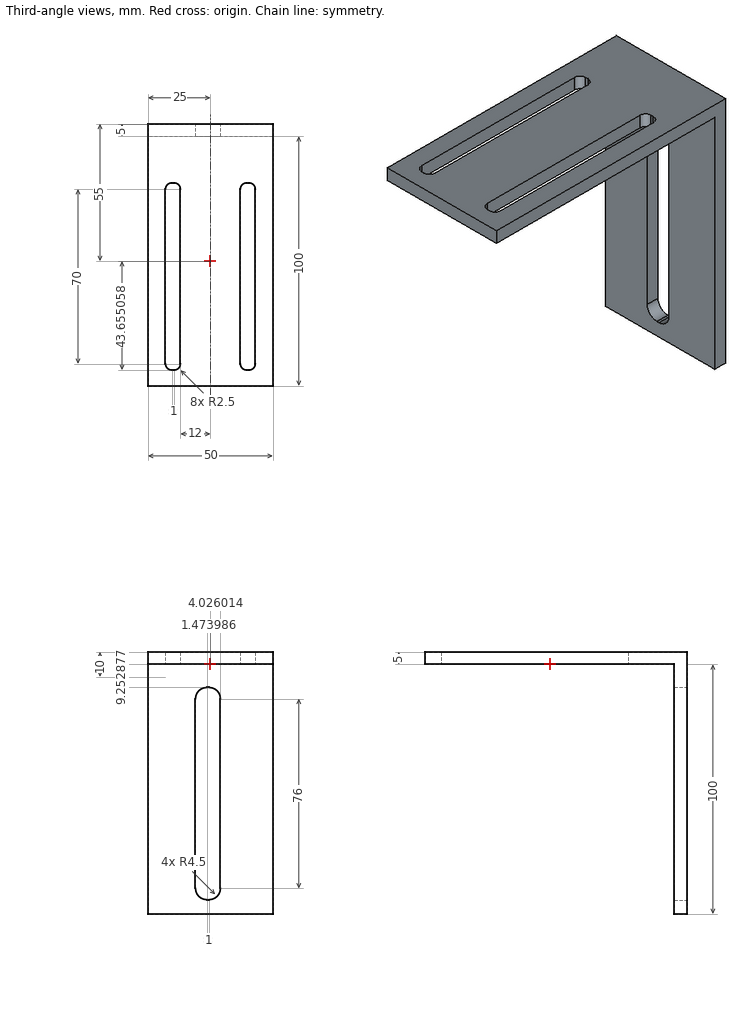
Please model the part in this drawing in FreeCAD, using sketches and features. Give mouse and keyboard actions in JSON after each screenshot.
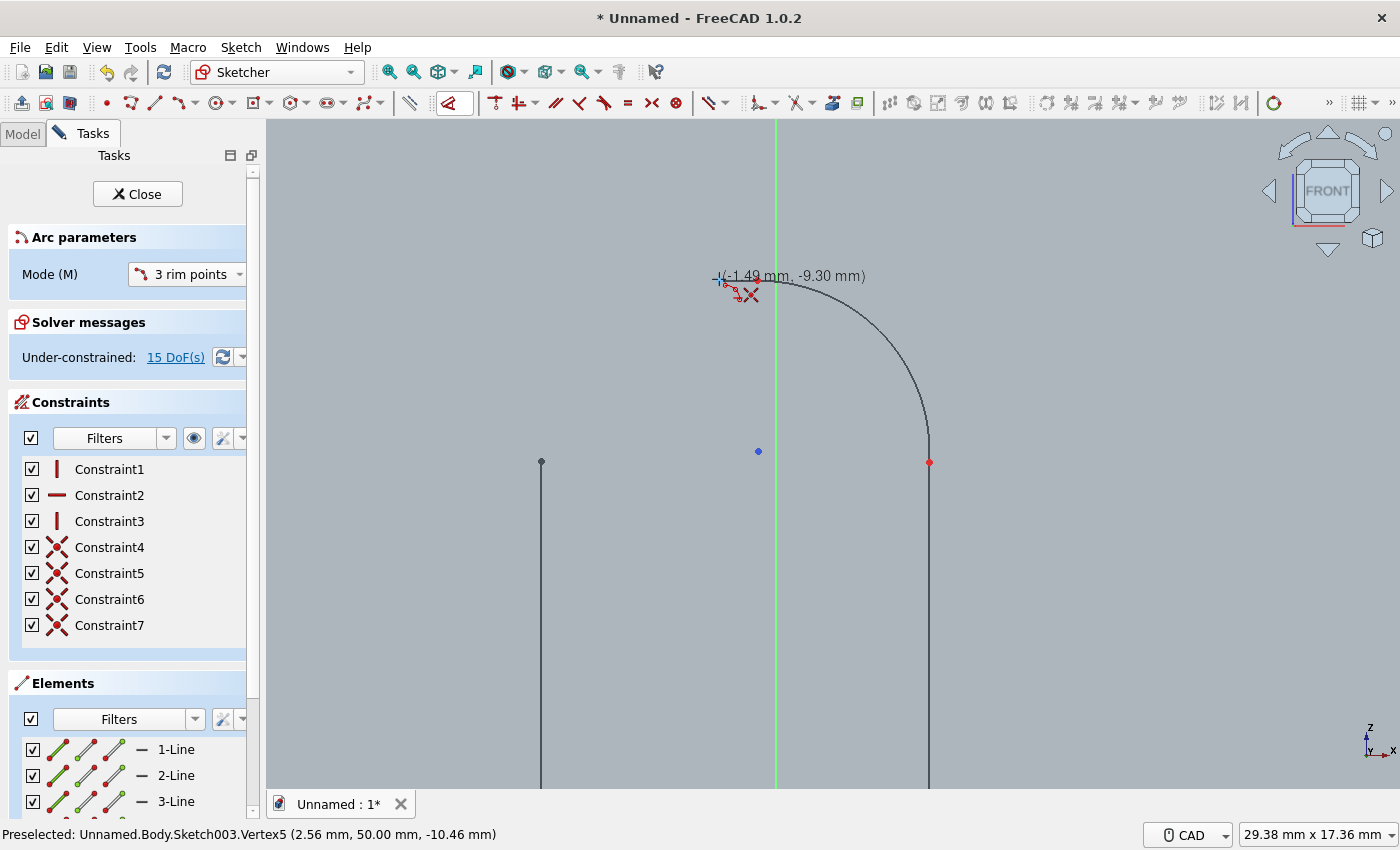
{"action": "left_click", "coordinate": [719, 281]}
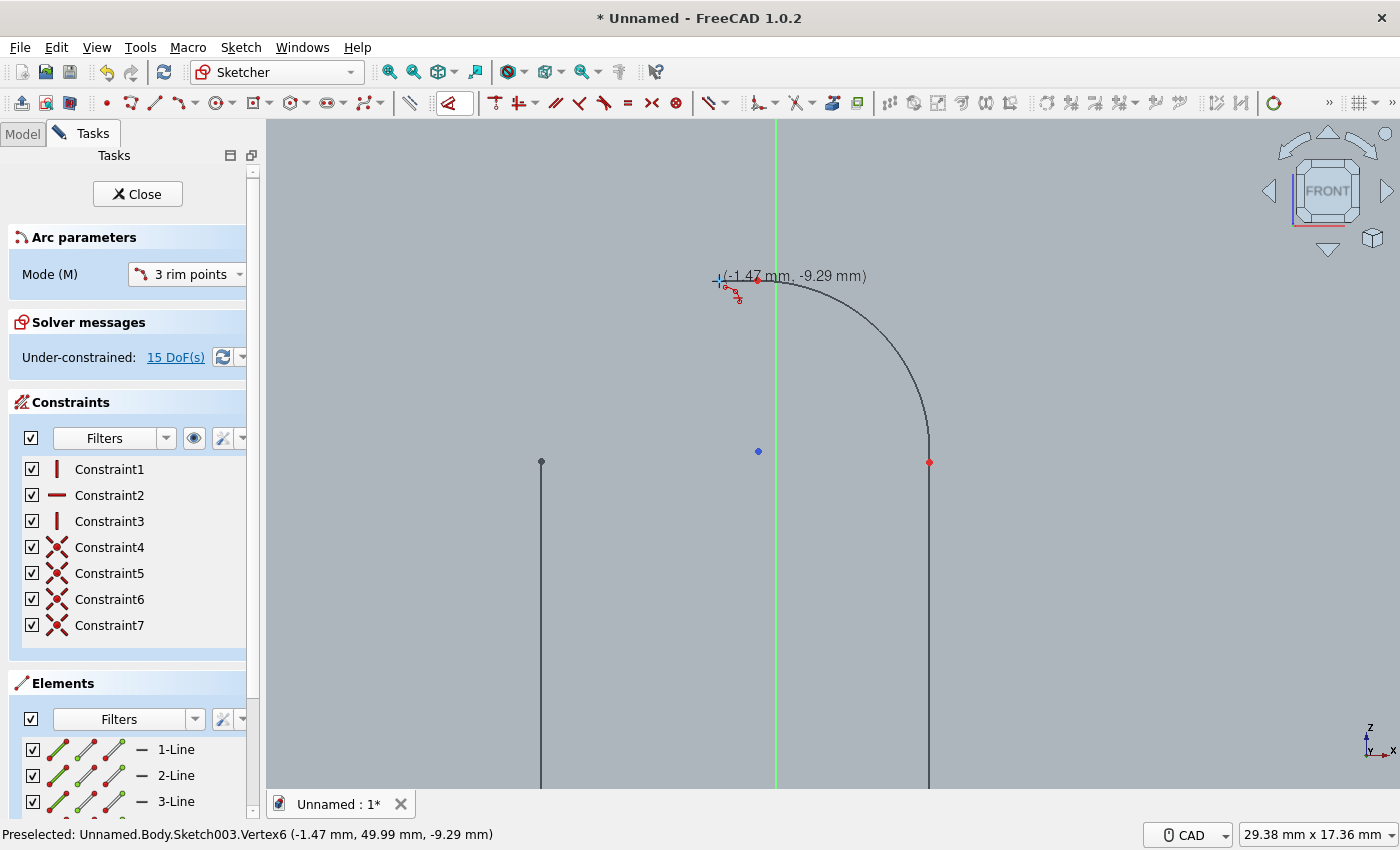
{"action": "scroll", "coordinate": [768, 294], "scroll_direction": "down", "scroll_amount": 11}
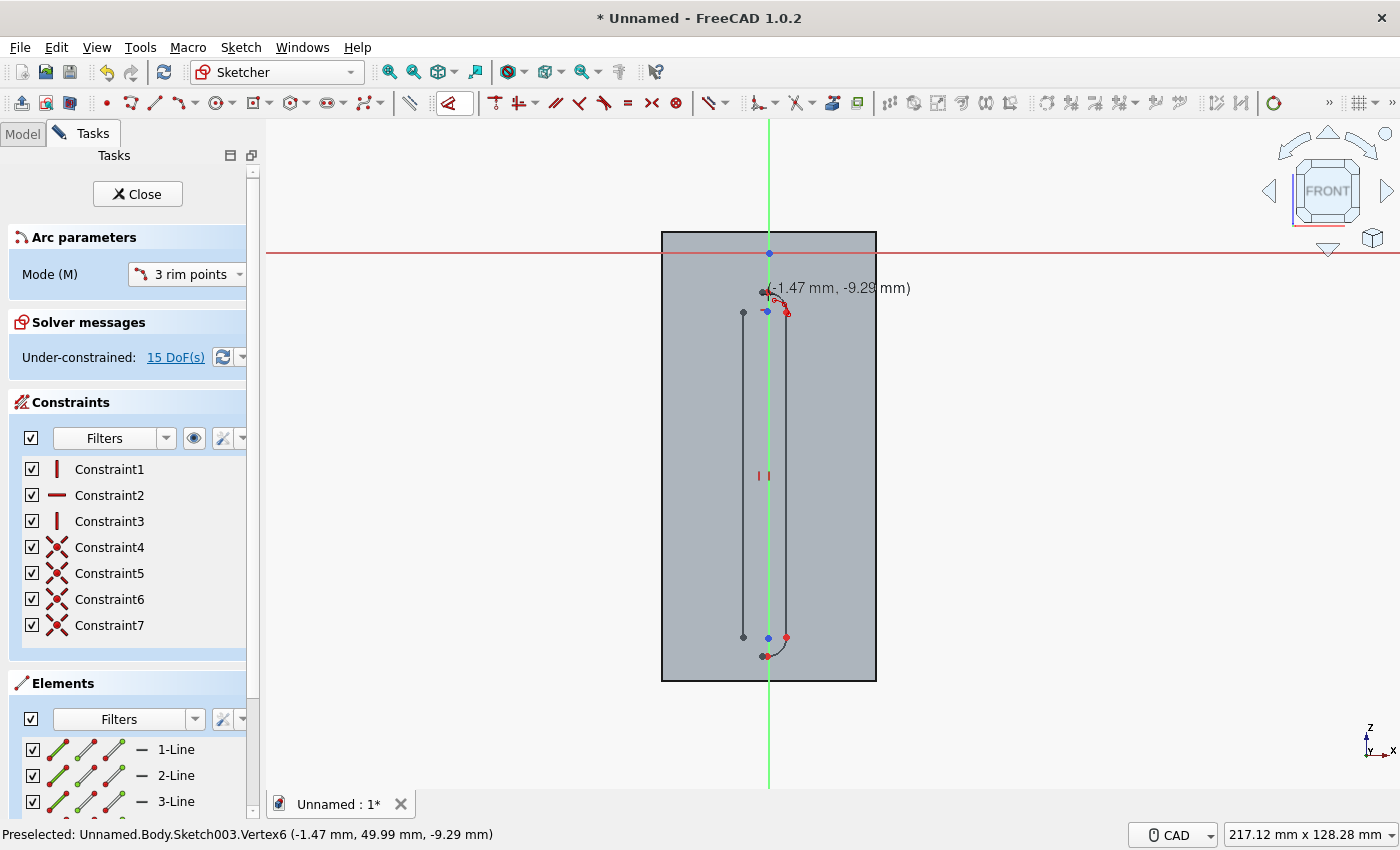
{"action": "left_click", "coordinate": [743, 313]}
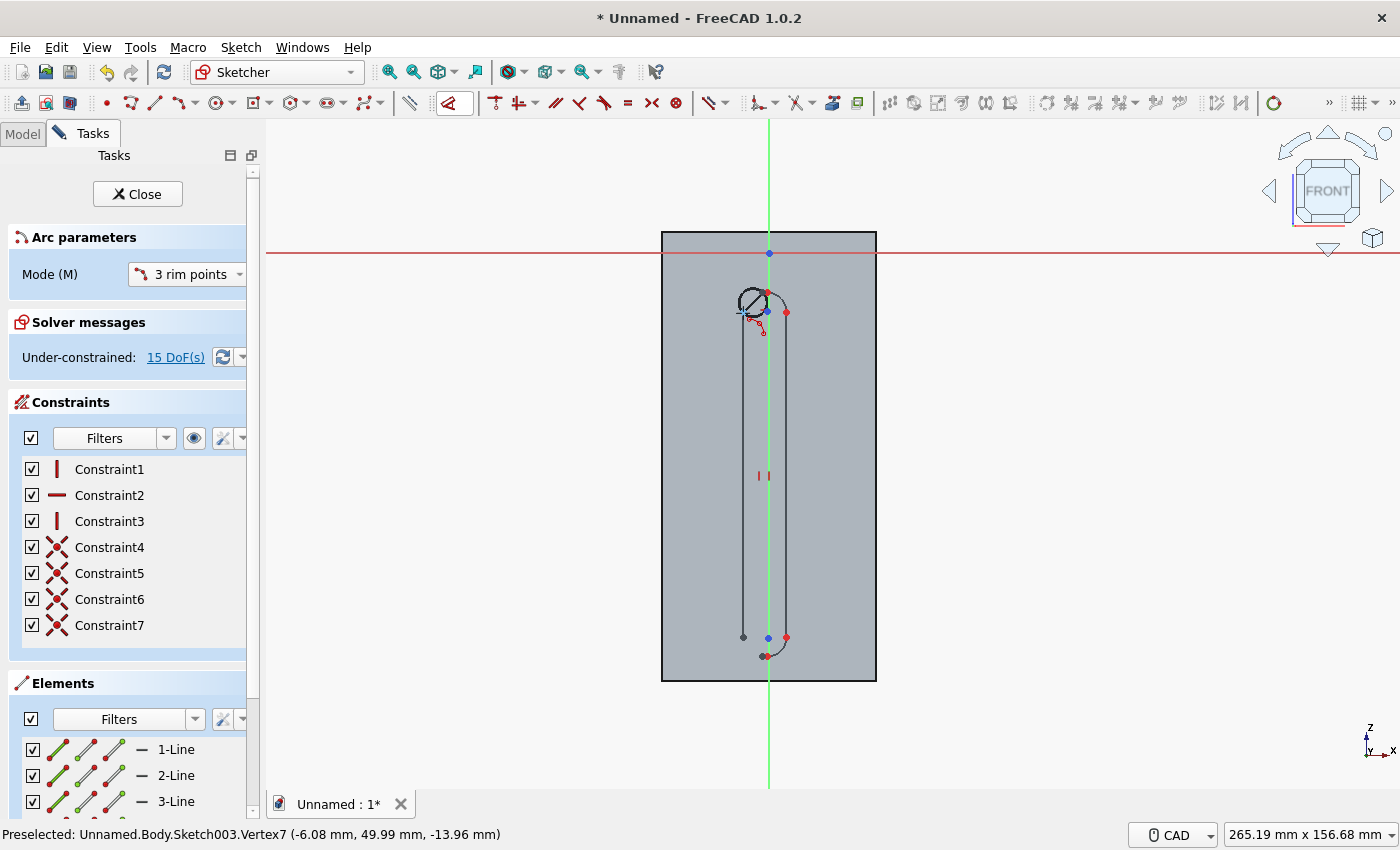
{"action": "scroll", "coordinate": [749, 298], "scroll_direction": "up", "scroll_amount": 6}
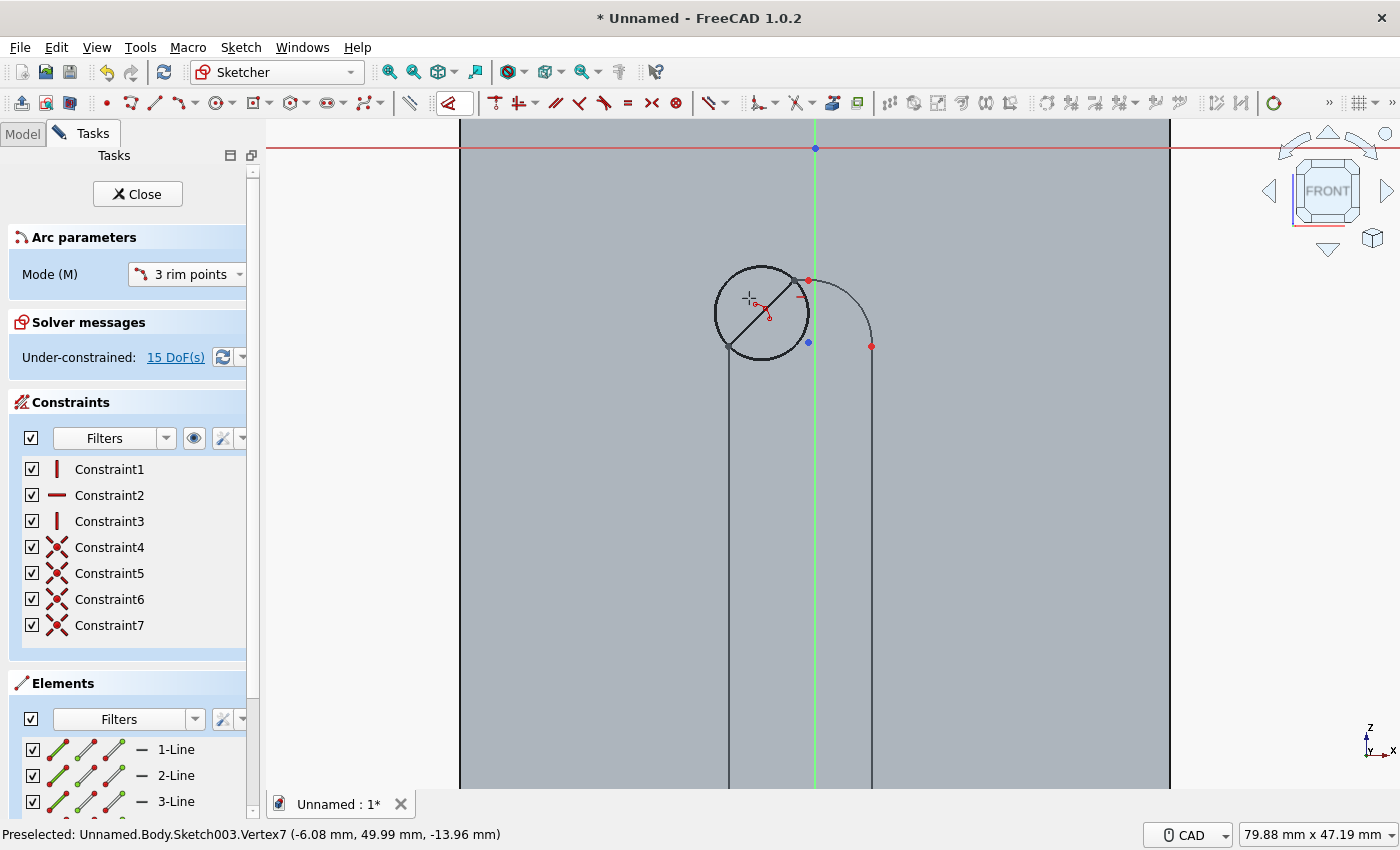
{"action": "left_click", "coordinate": [749, 298]}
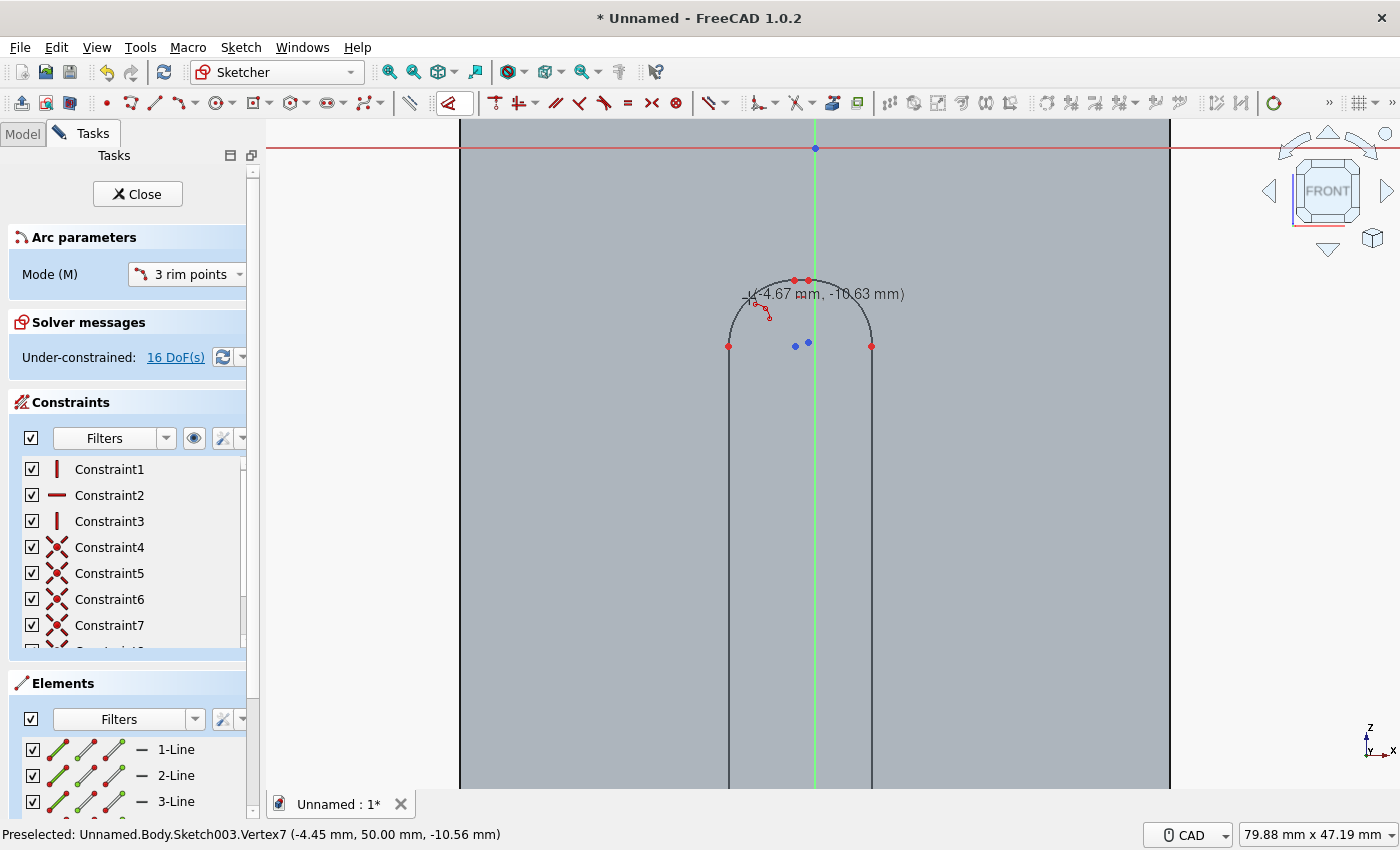
{"action": "scroll", "coordinate": [749, 297], "scroll_direction": "down", "scroll_amount": 6}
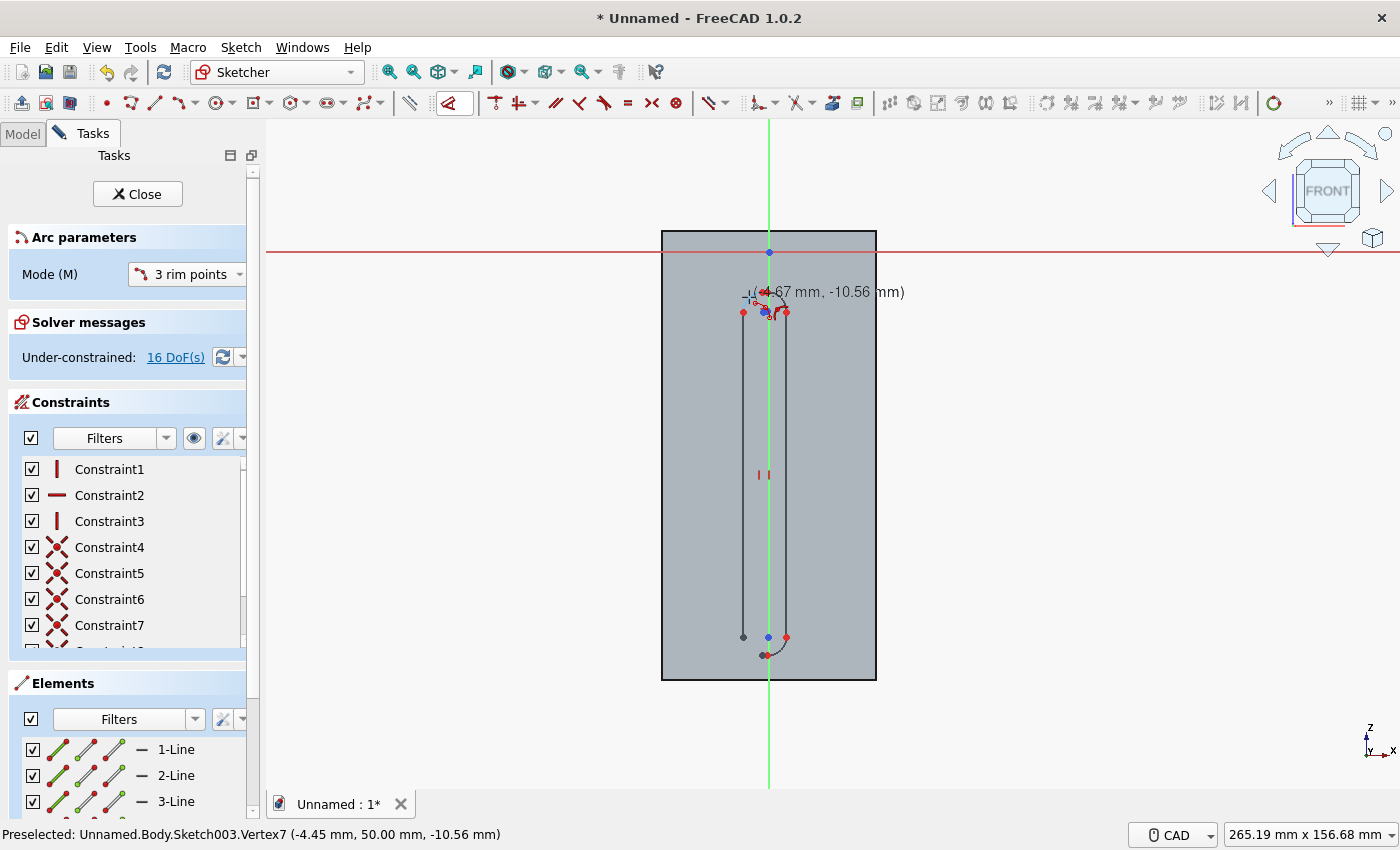
{"action": "left_click", "coordinate": [743, 637]}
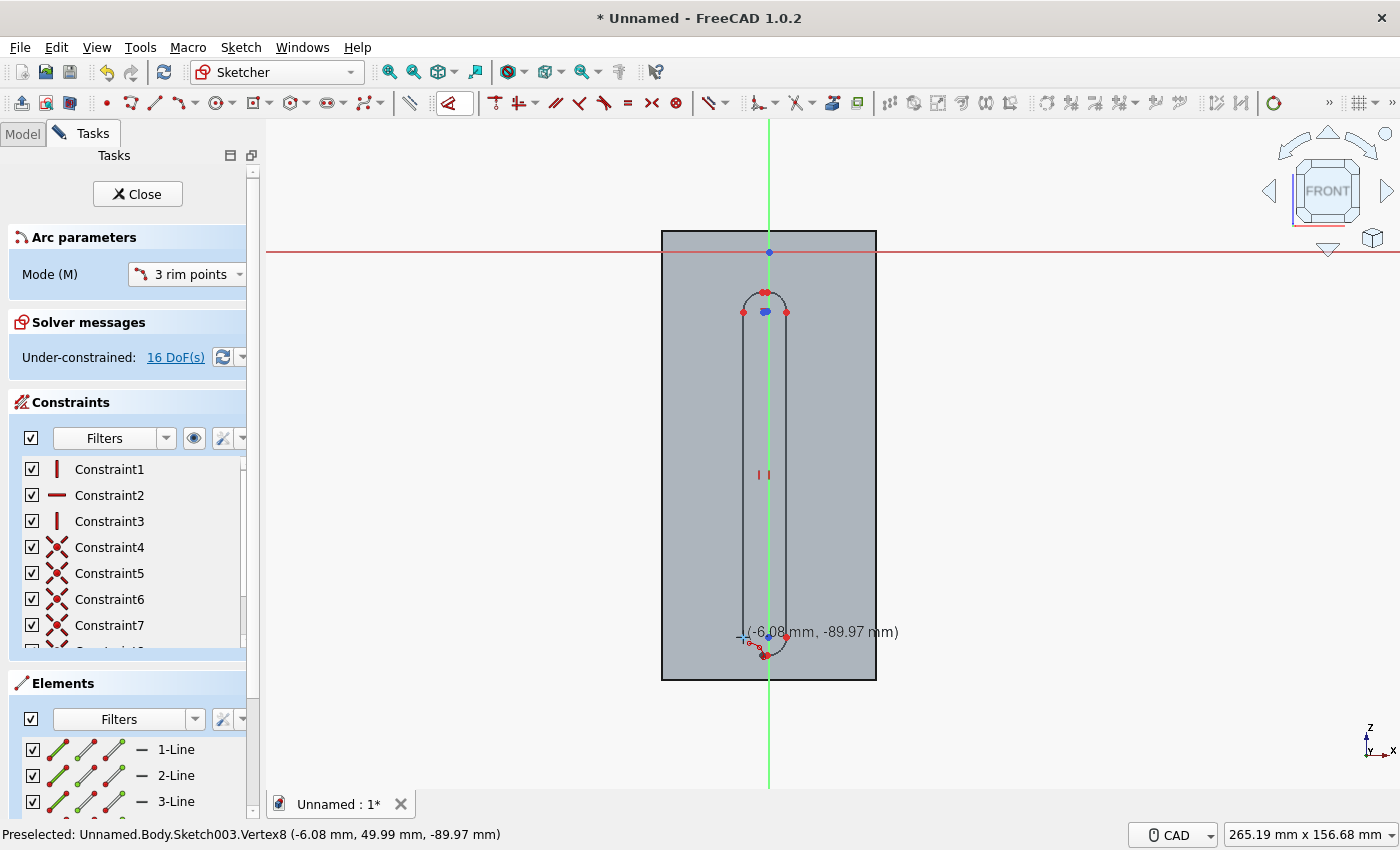
{"action": "scroll", "coordinate": [763, 655], "scroll_direction": "up", "scroll_amount": 11}